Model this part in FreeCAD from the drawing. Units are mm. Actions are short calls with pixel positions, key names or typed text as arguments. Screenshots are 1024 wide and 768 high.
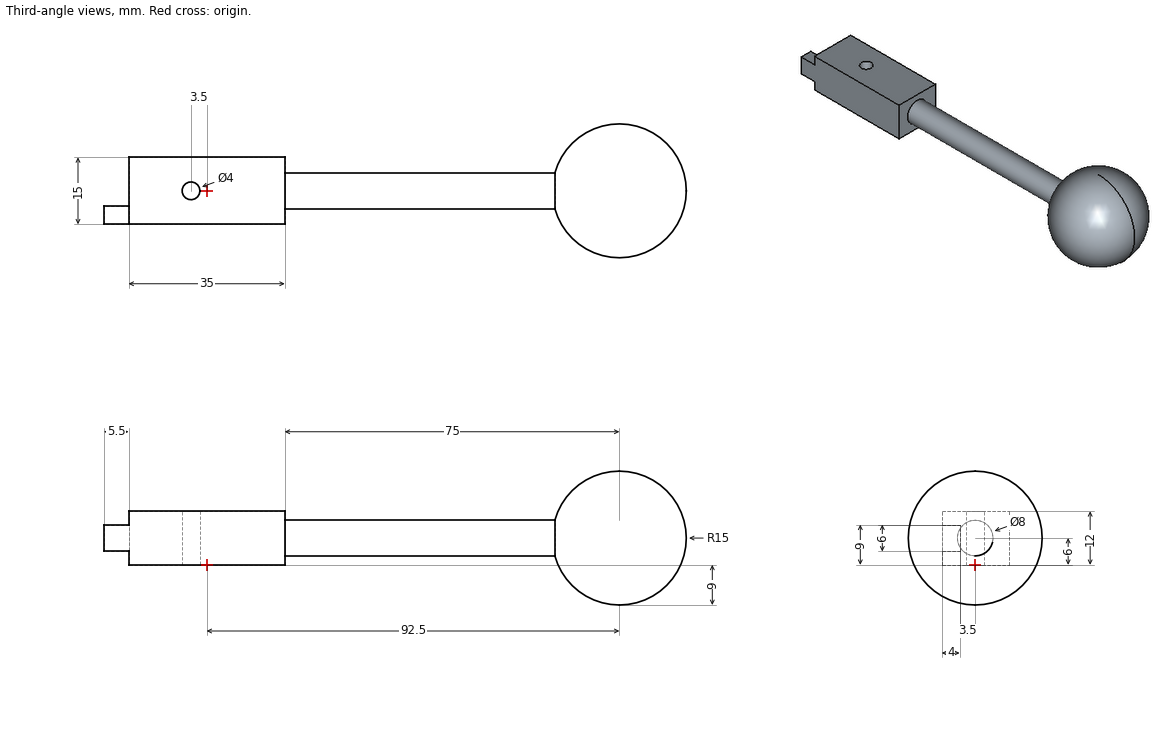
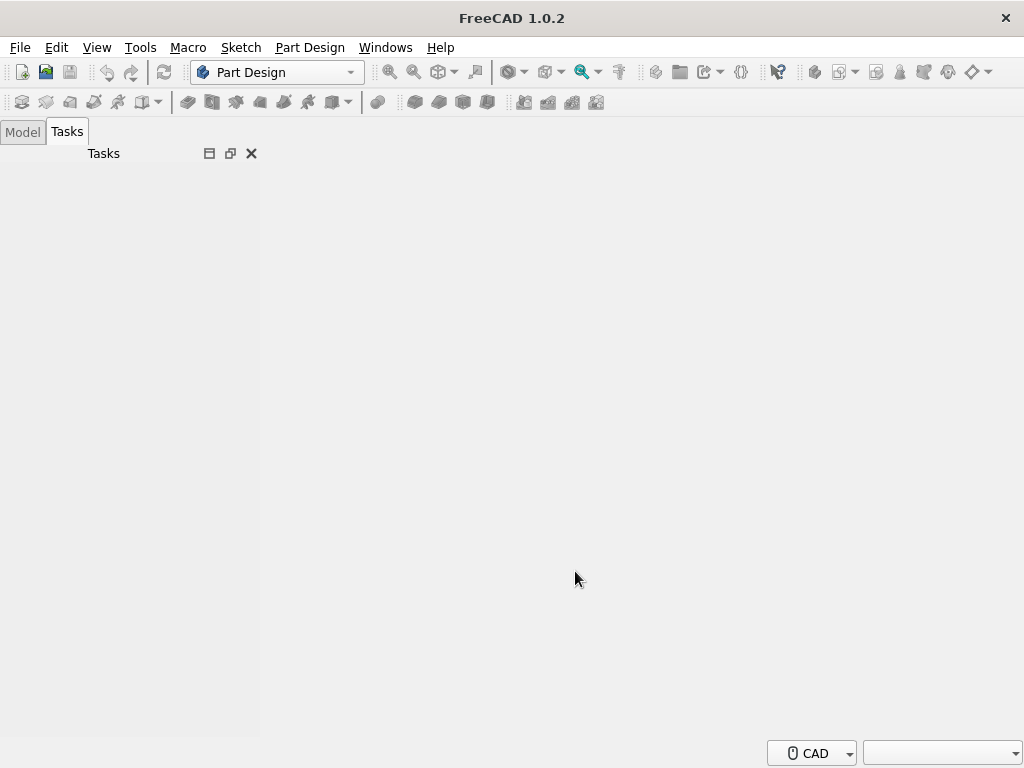
click(22, 72)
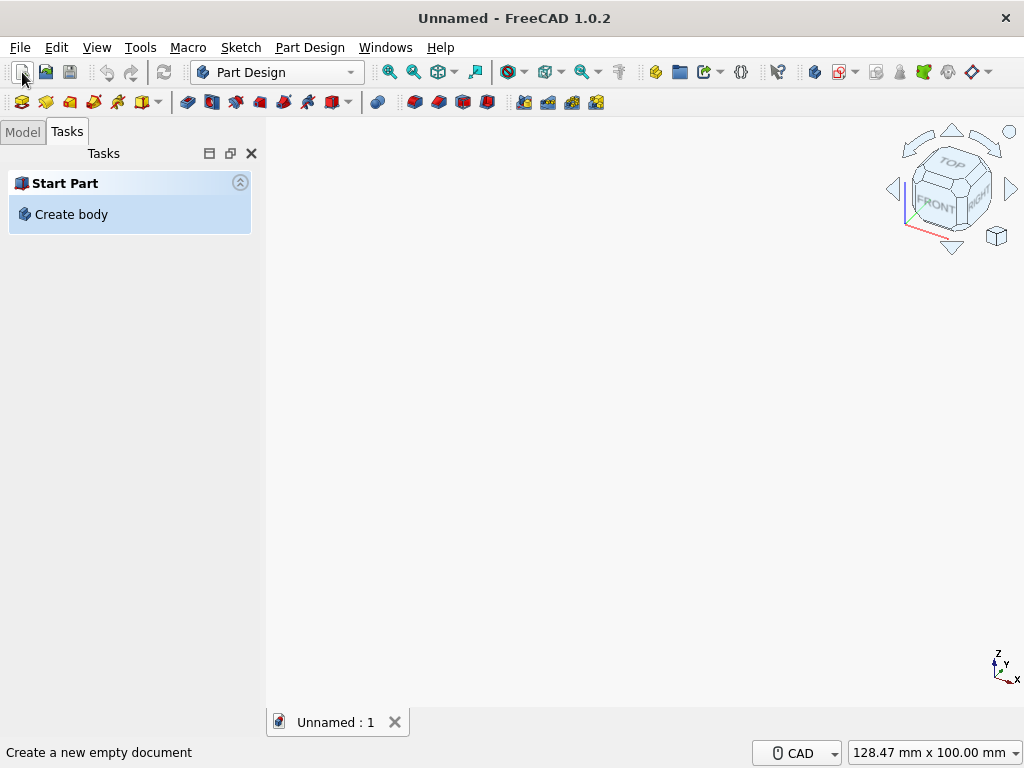
click(840, 72)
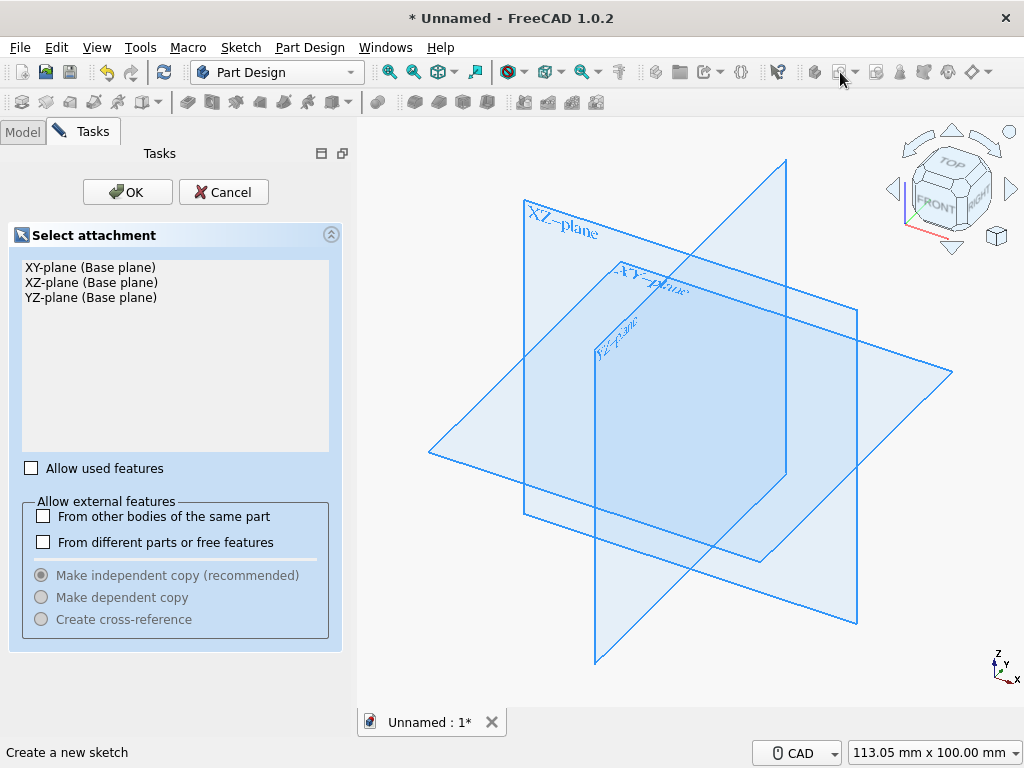
click(82, 268)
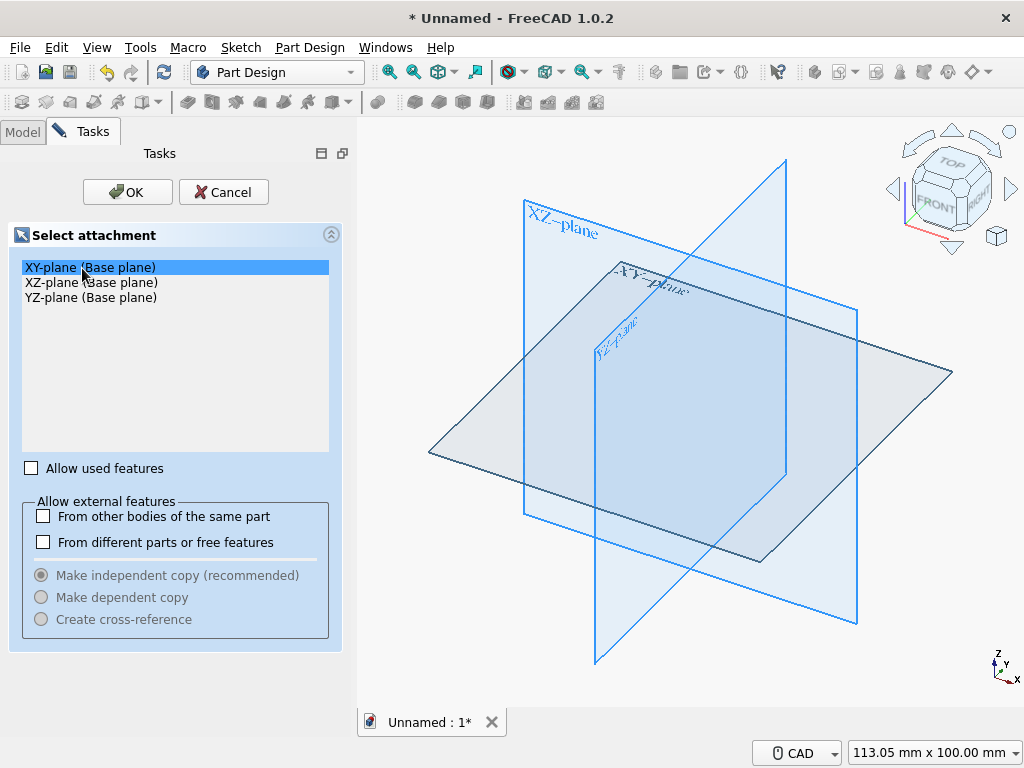
click(128, 192)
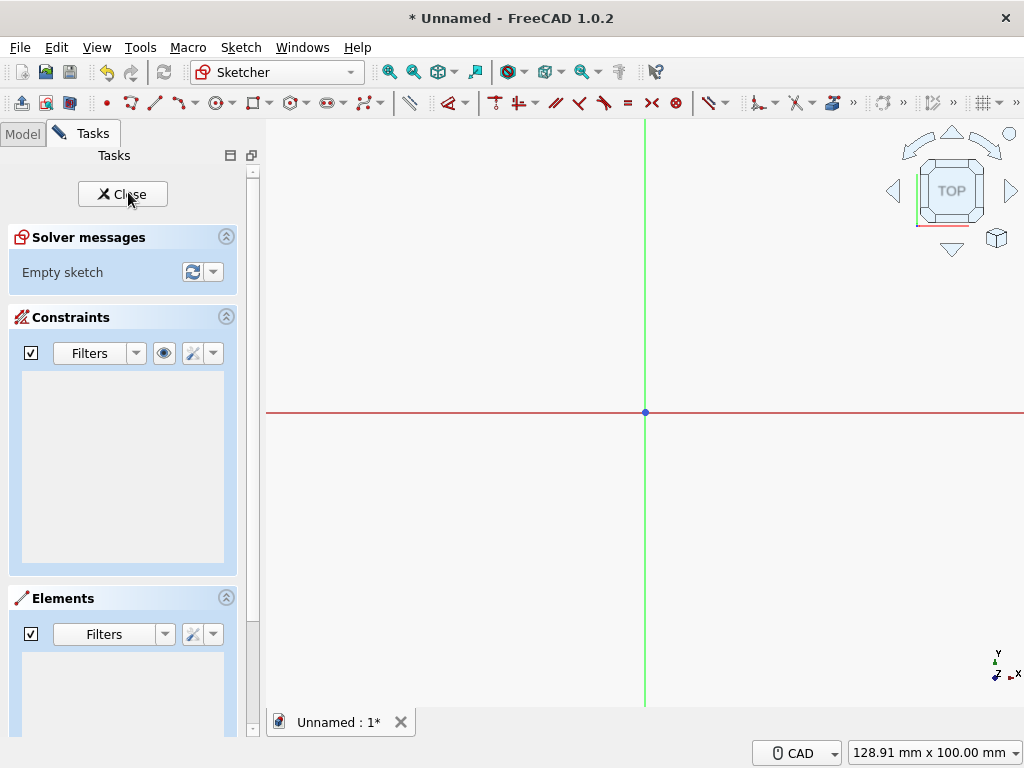
scroll(728, 413, up, 3)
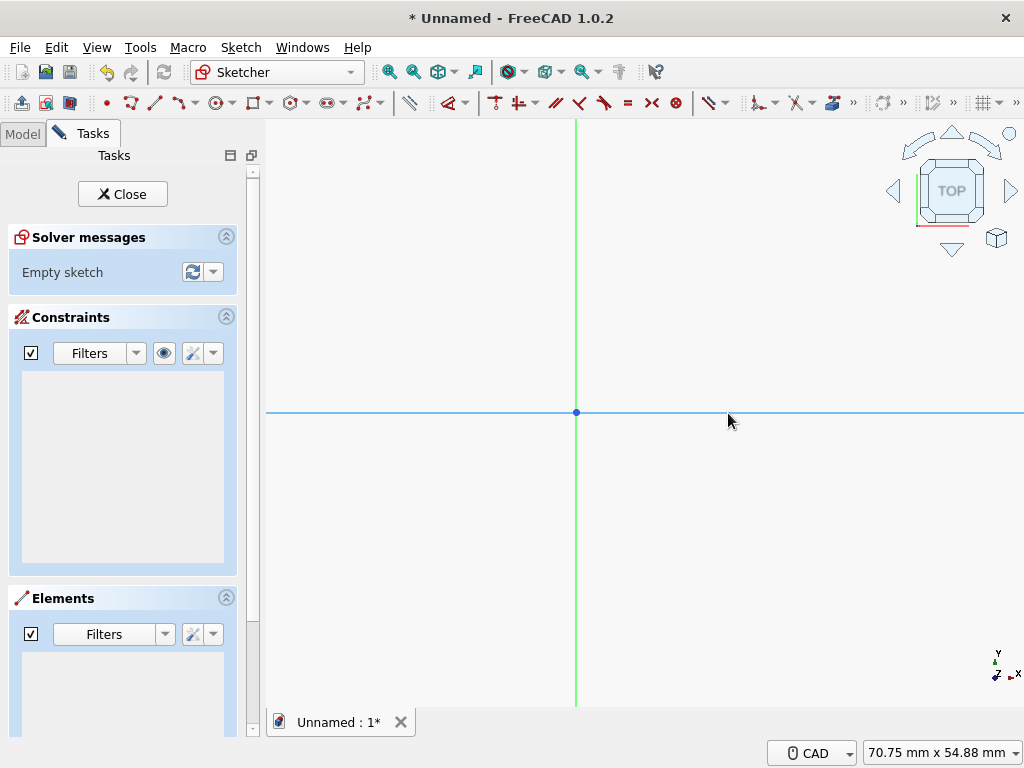
click(272, 104)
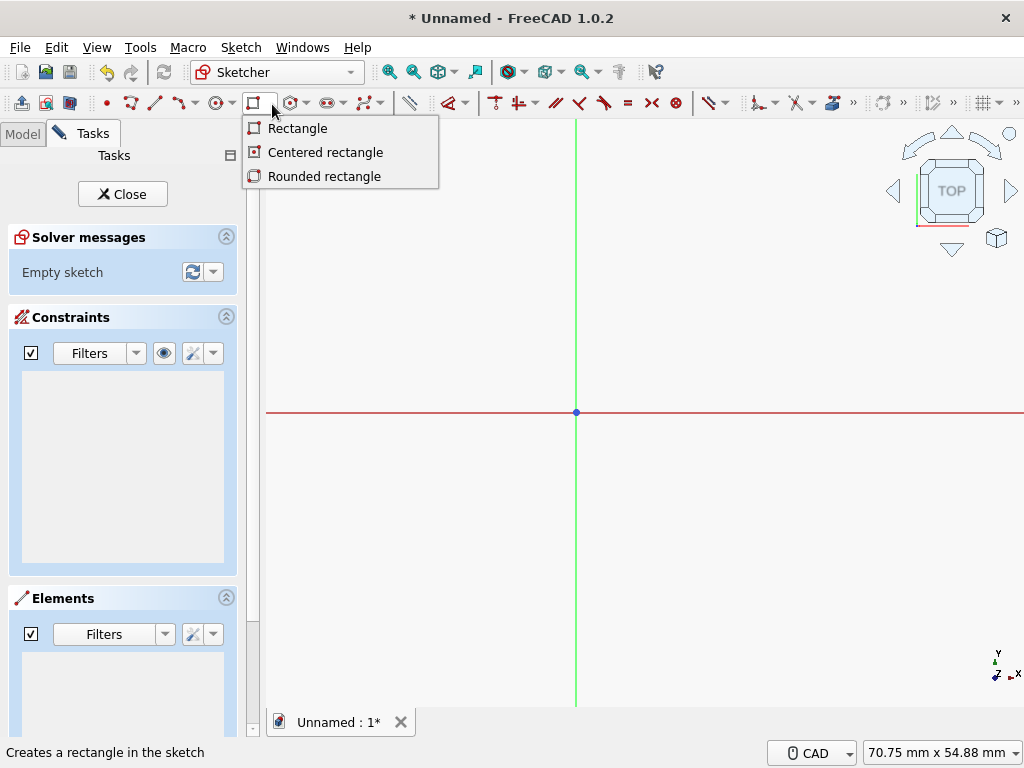
click(340, 152)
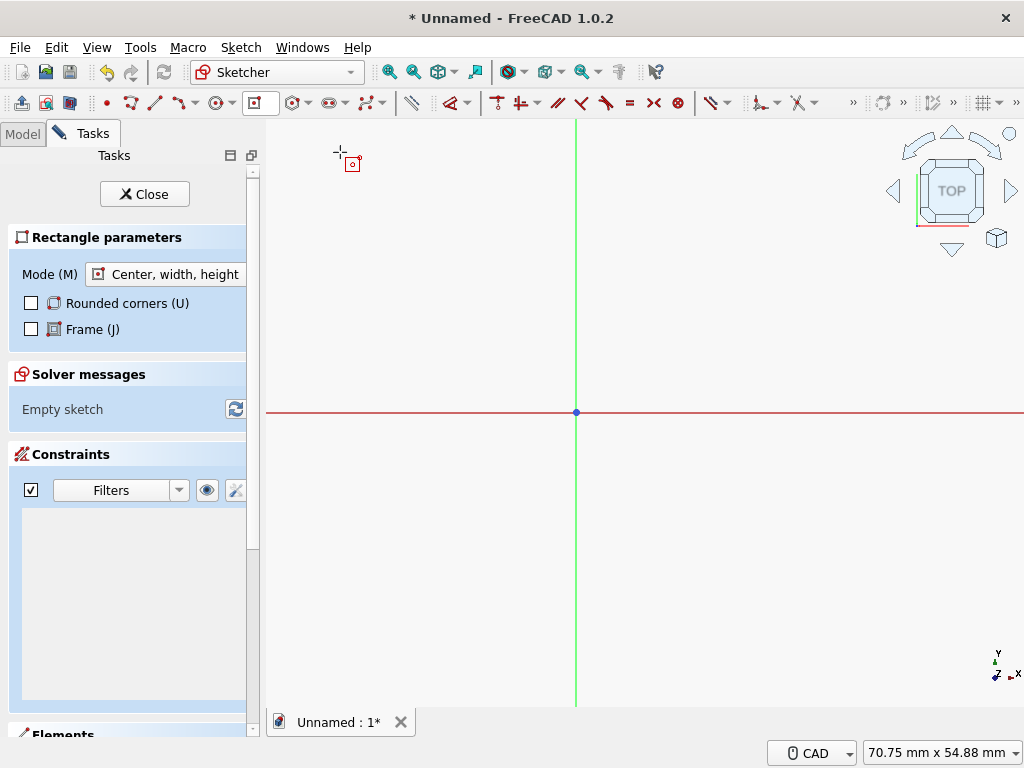
click(576, 413)
click(764, 332)
key(Escape)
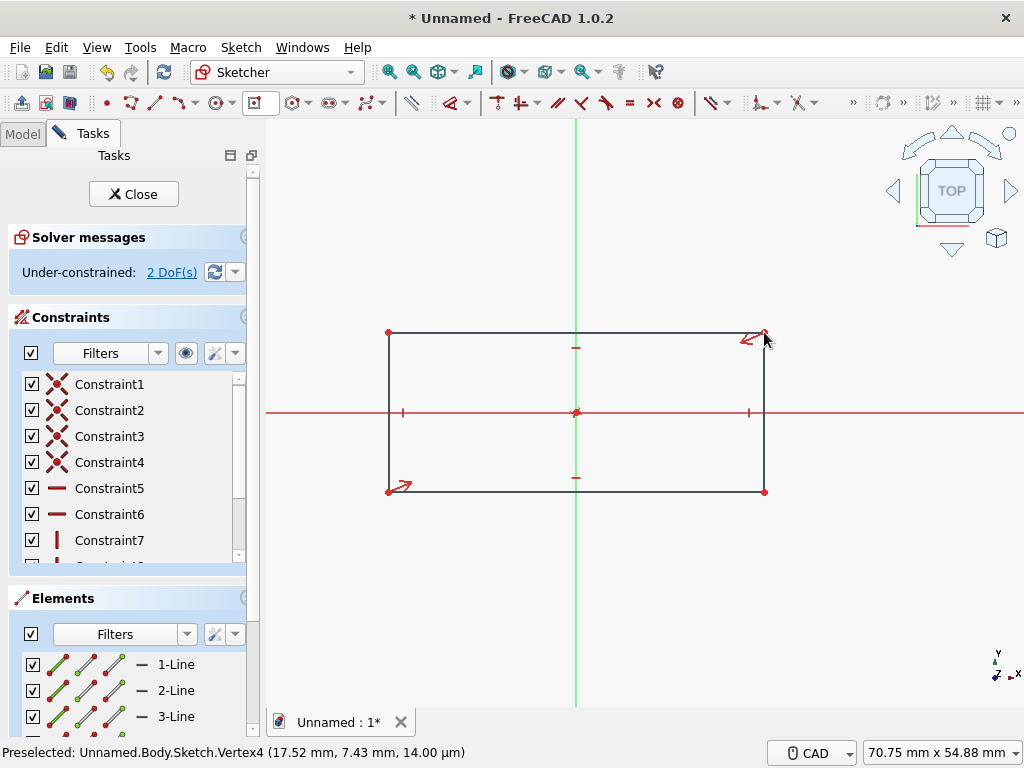
click(450, 104)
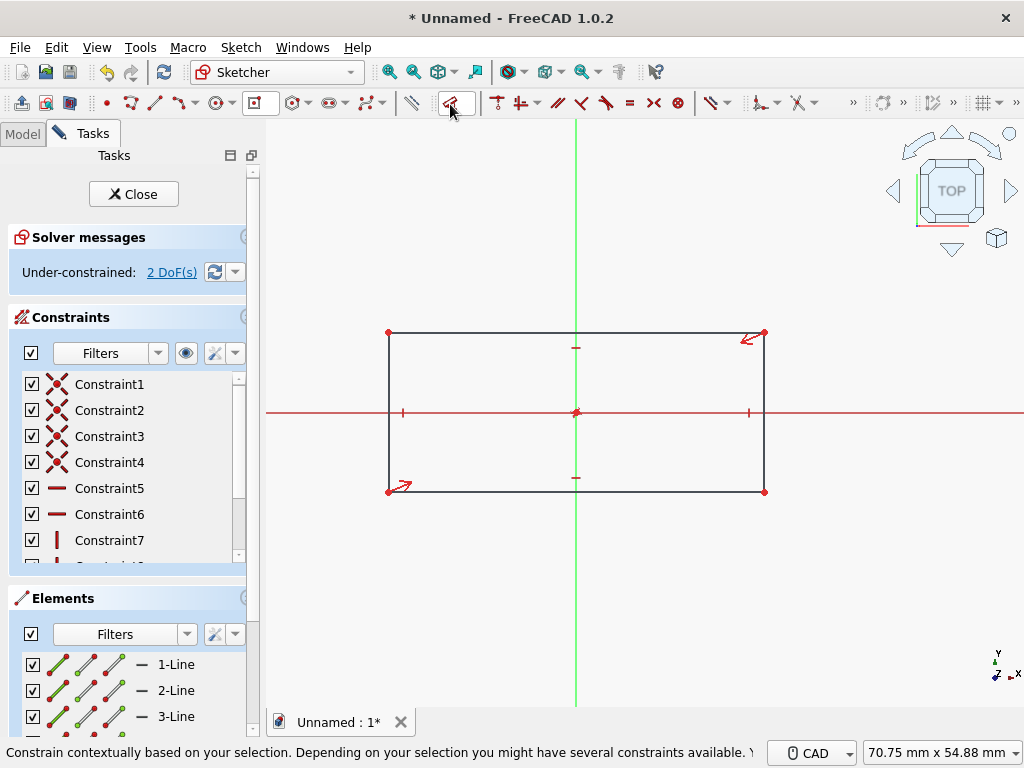
click(501, 492)
click(490, 526)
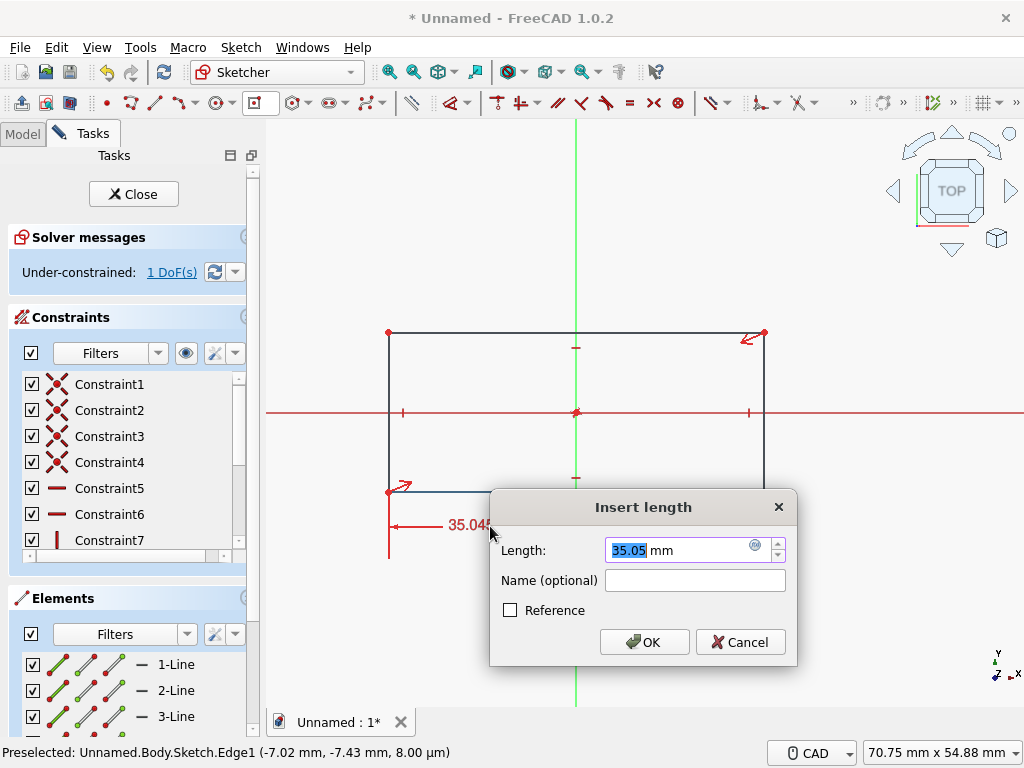
text(35)
key(Return)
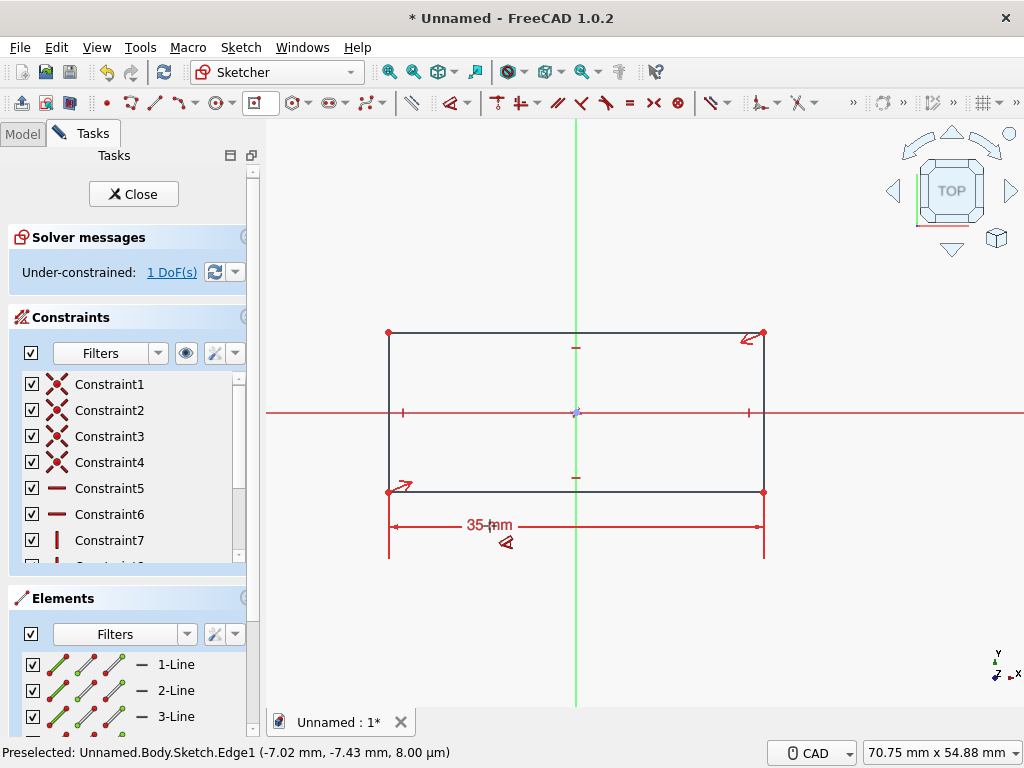
click(764, 444)
click(798, 376)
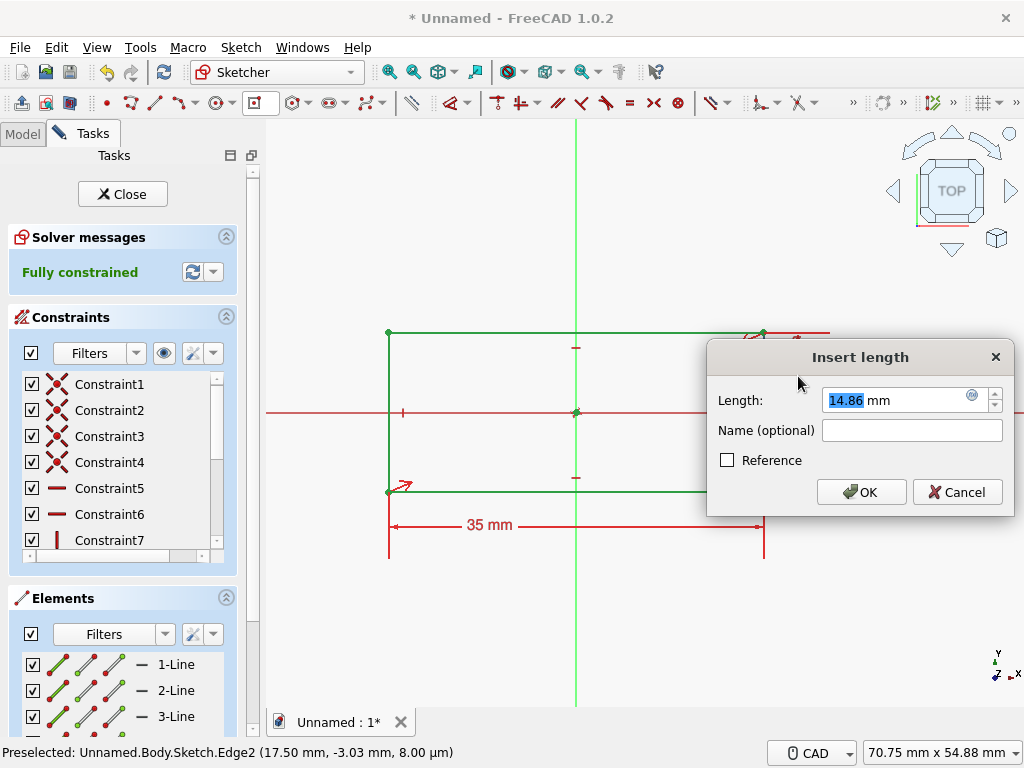
text(15)
key(Return)
key(Escape)